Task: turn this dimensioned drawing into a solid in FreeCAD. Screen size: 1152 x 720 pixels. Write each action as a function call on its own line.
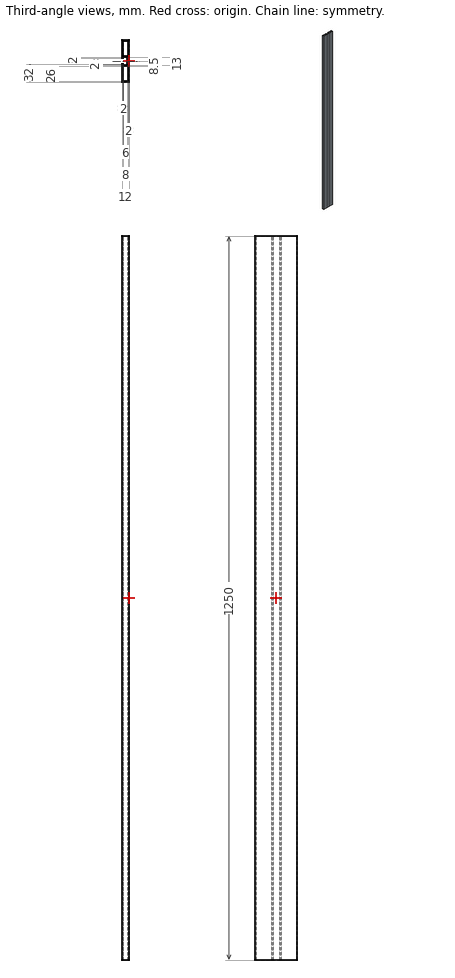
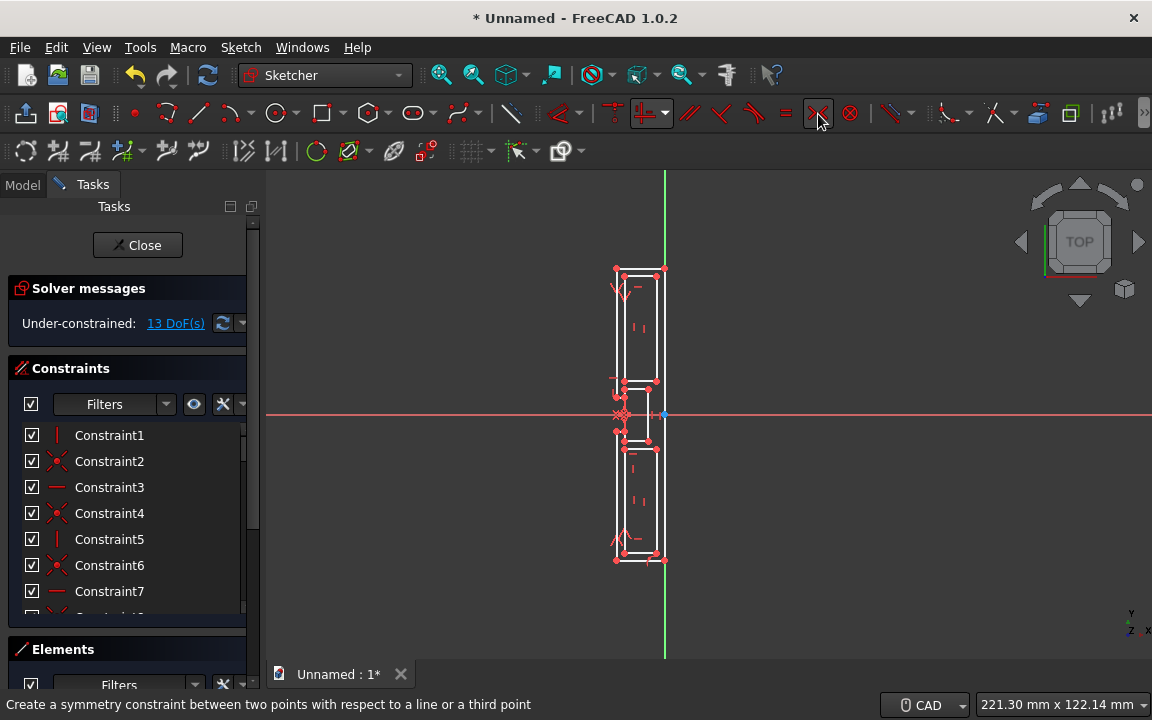
click(657, 449)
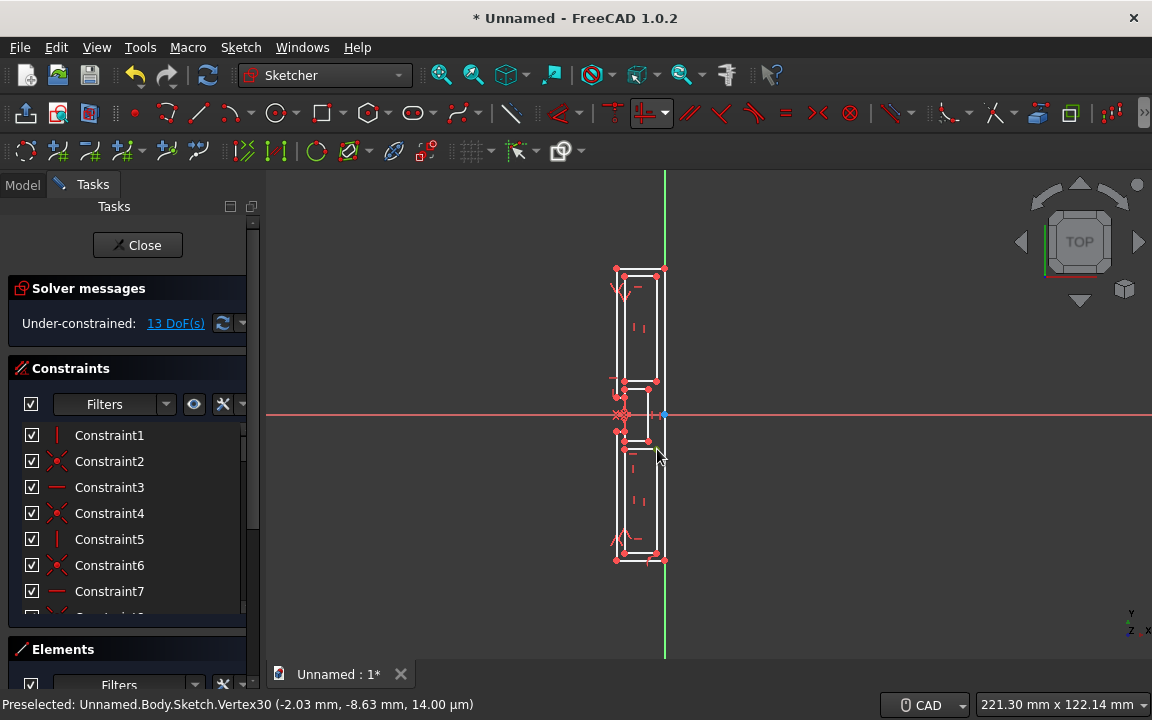
click(657, 381)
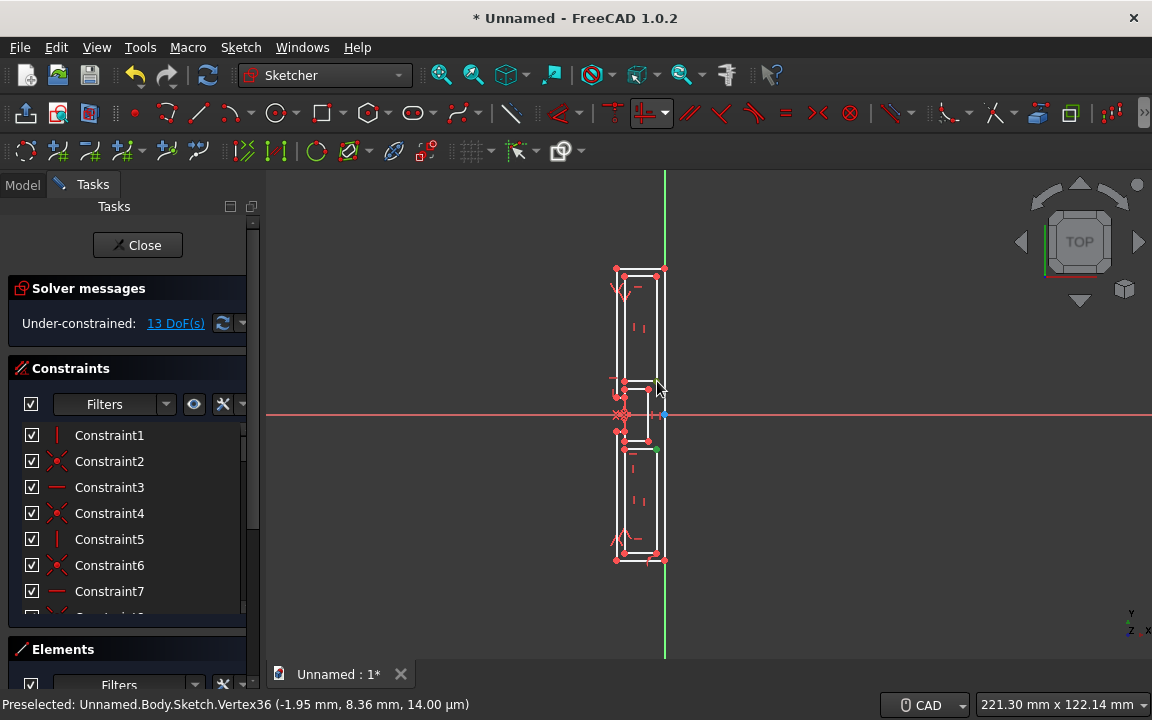
click(344, 415)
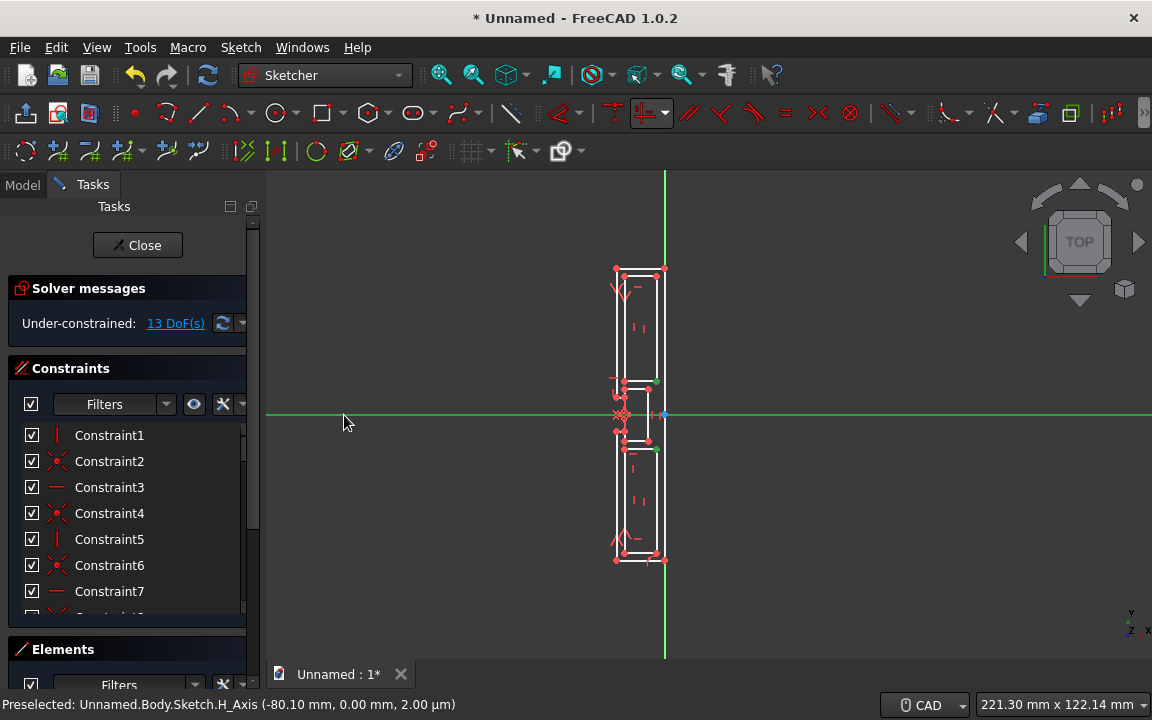
click(818, 114)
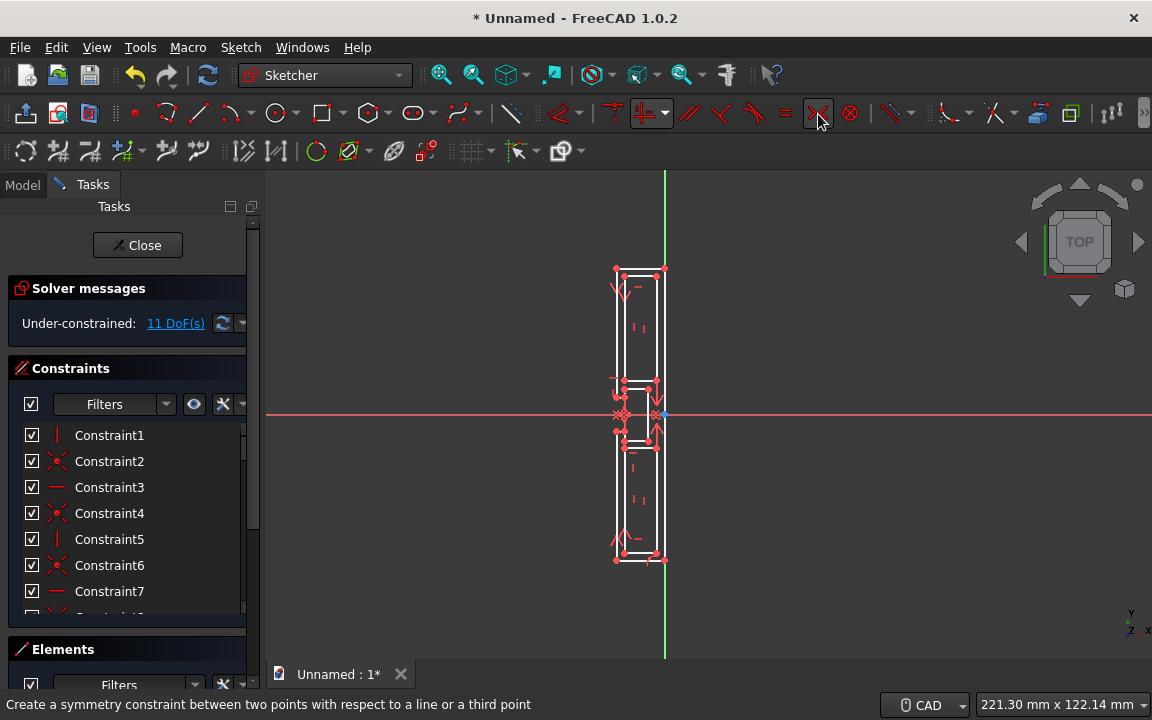
click(558, 114)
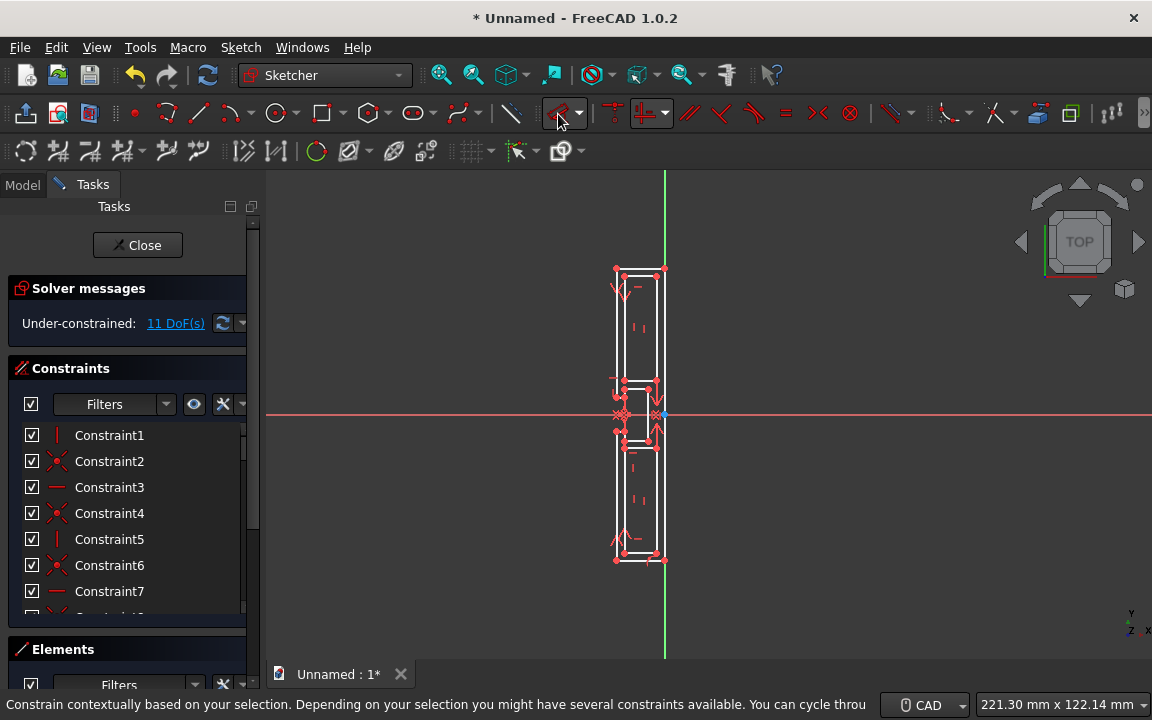
scroll(641, 441, up, 4)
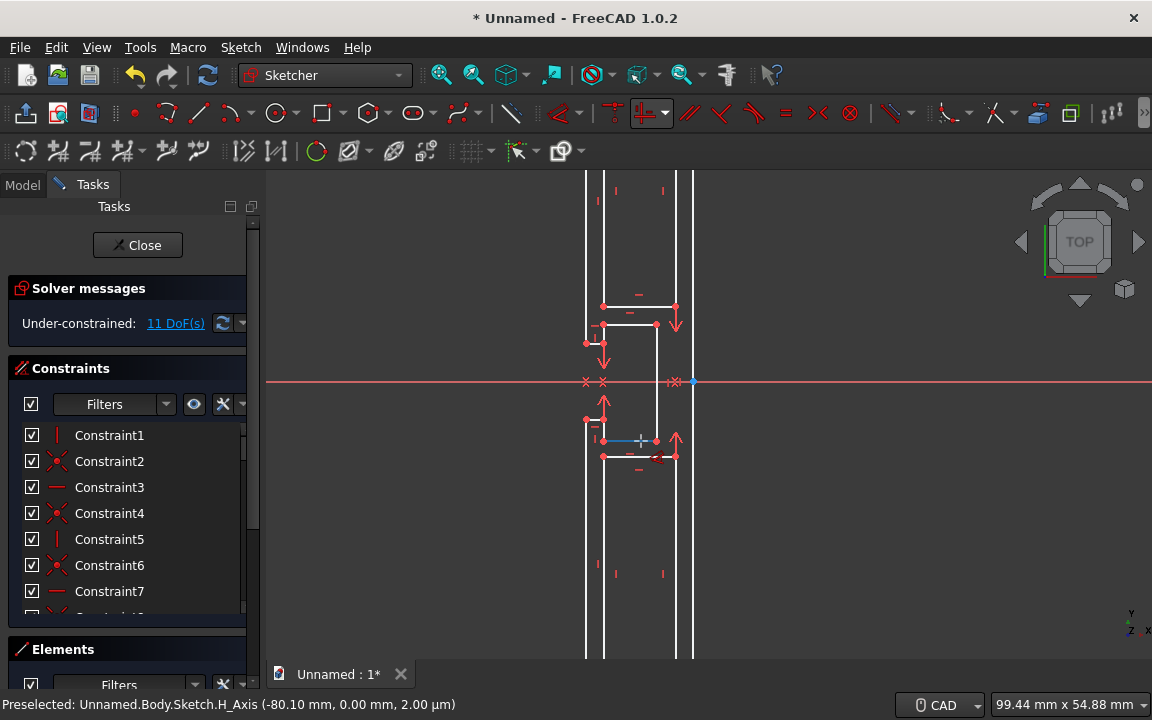
click(641, 441)
click(630, 475)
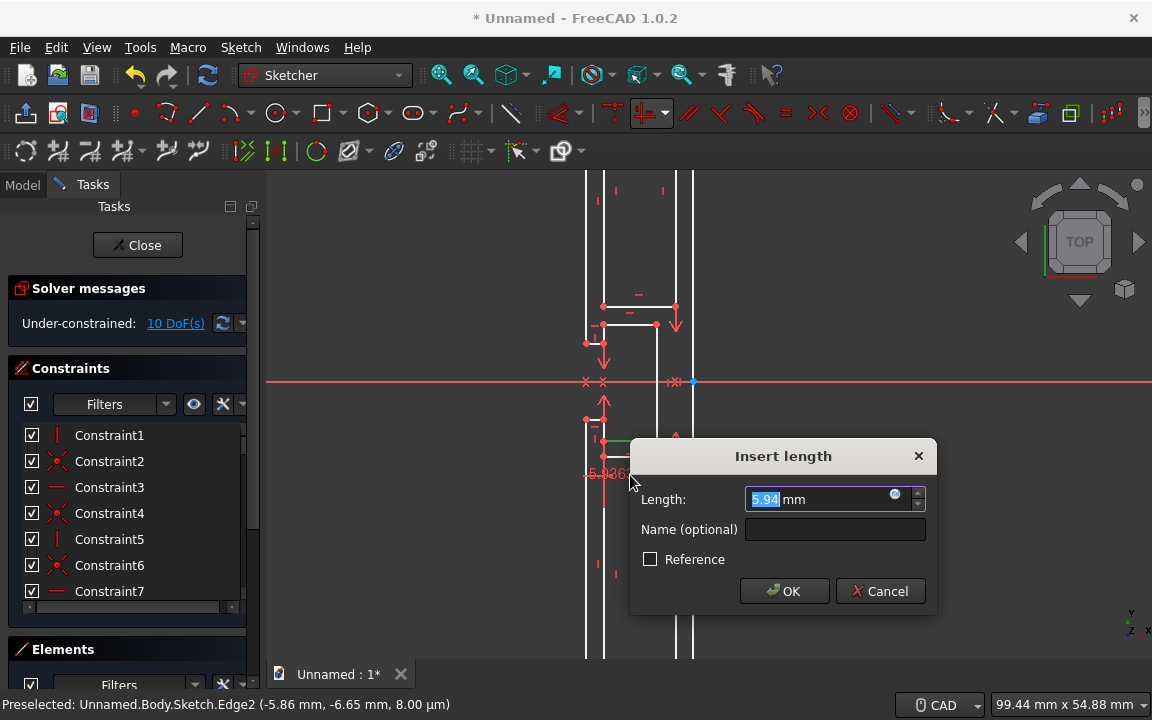
text(6)
key(Return)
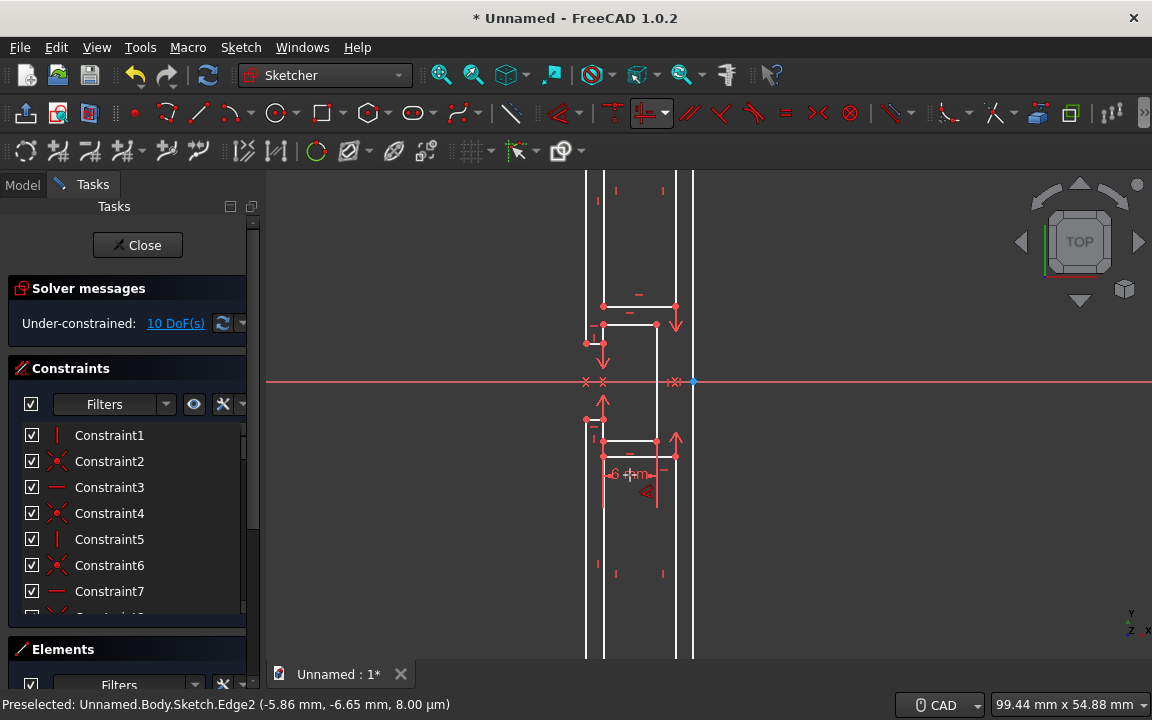
scroll(603, 431, up, 5)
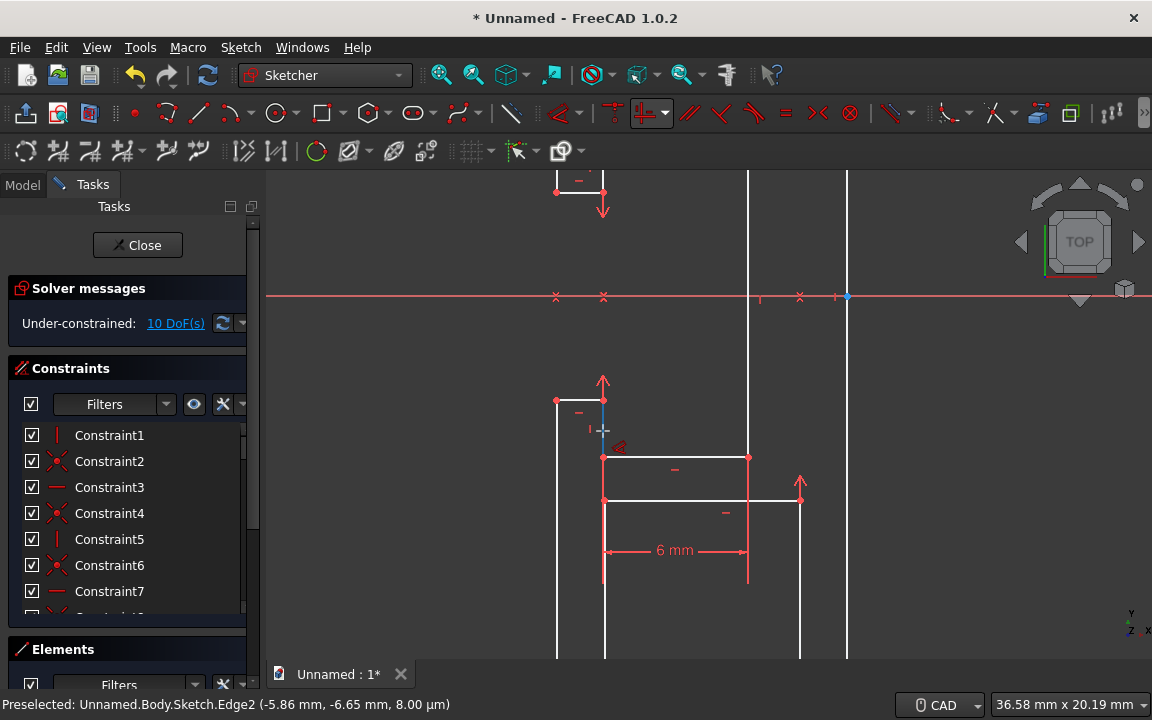
click(603, 429)
click(637, 429)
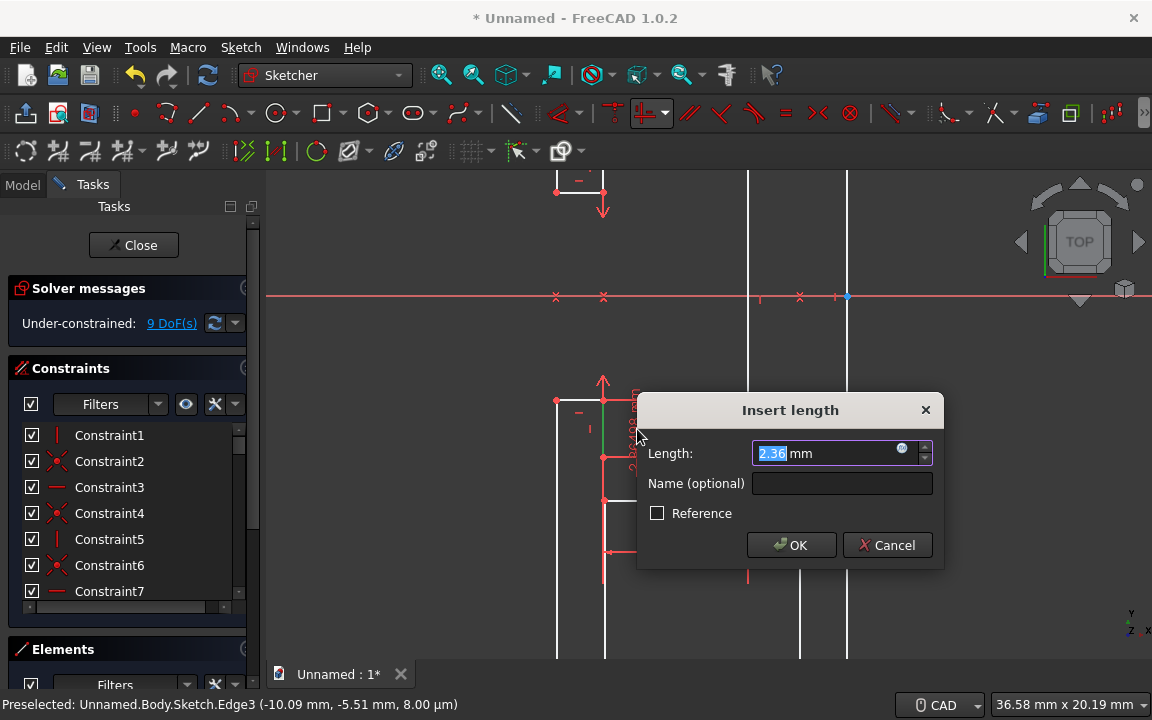
text(2)
key(Return)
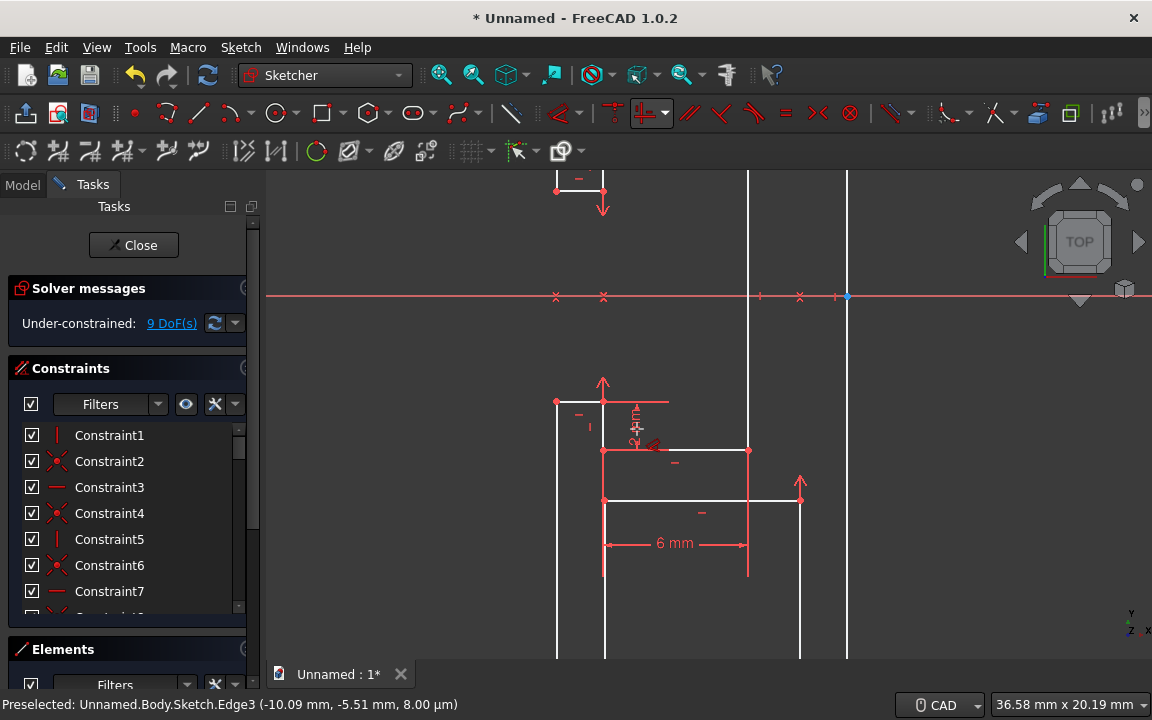
click(589, 402)
click(580, 368)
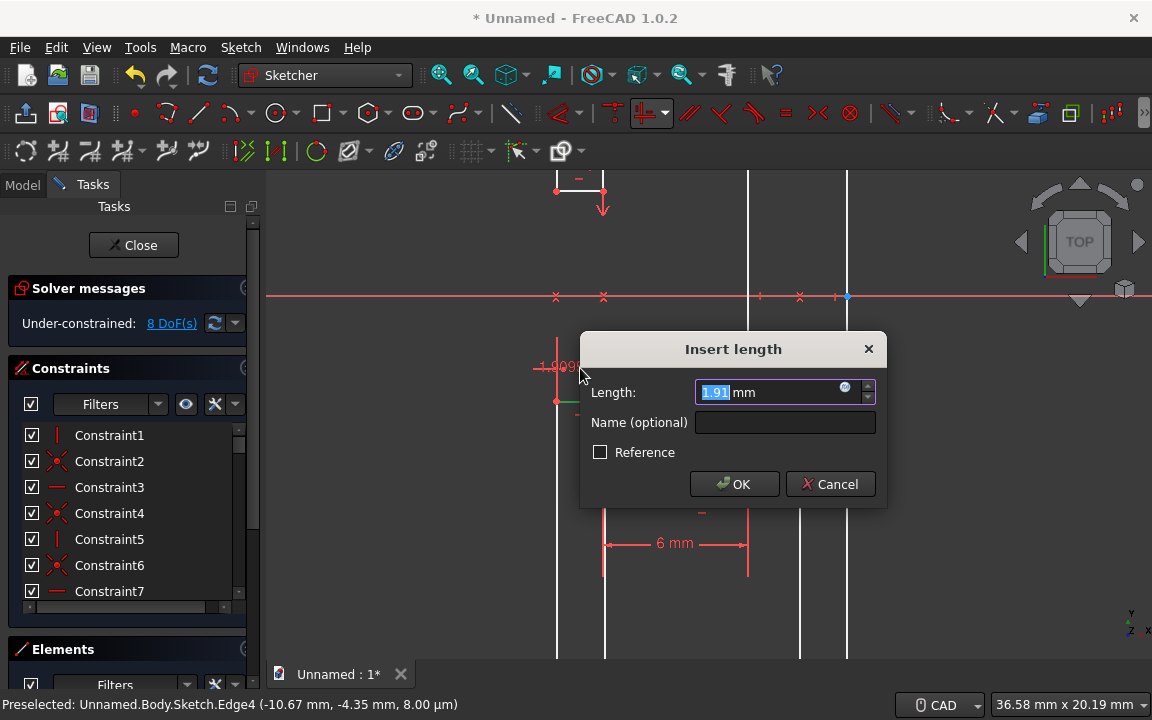
text(2)
key(Return)